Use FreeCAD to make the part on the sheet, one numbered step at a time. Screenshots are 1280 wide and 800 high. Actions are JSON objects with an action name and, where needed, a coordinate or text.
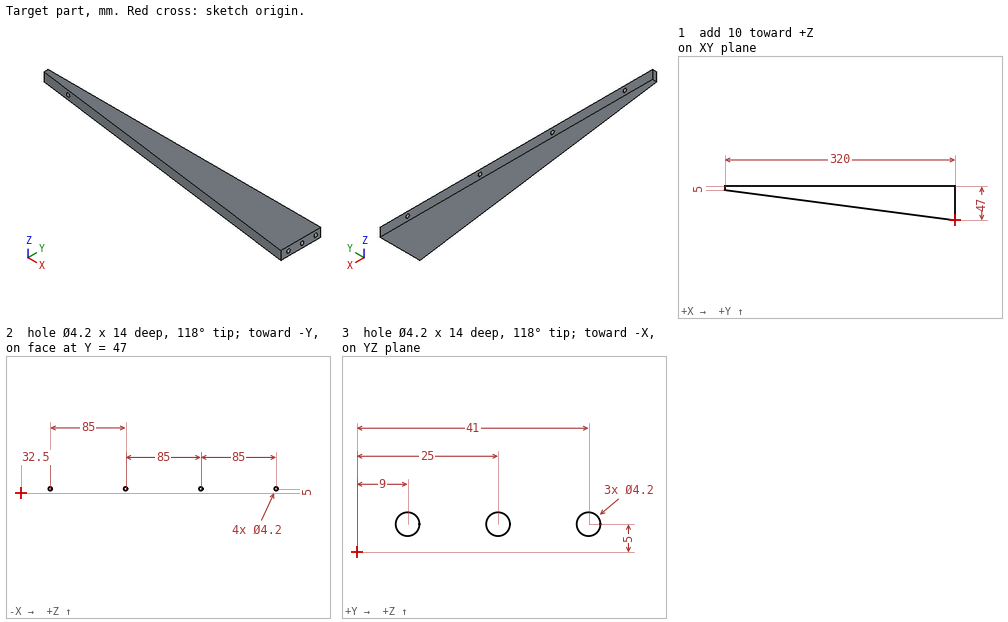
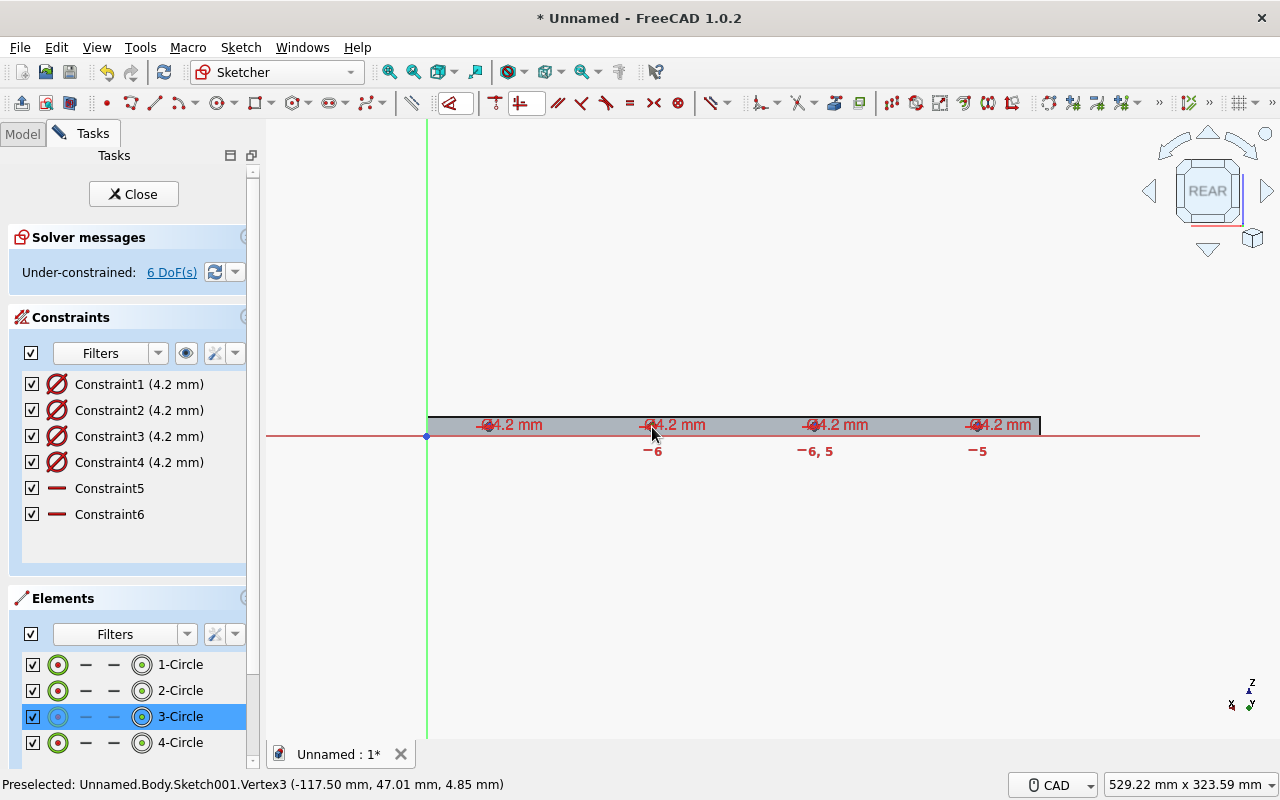
{"action": "left_click", "coordinate": [489, 427]}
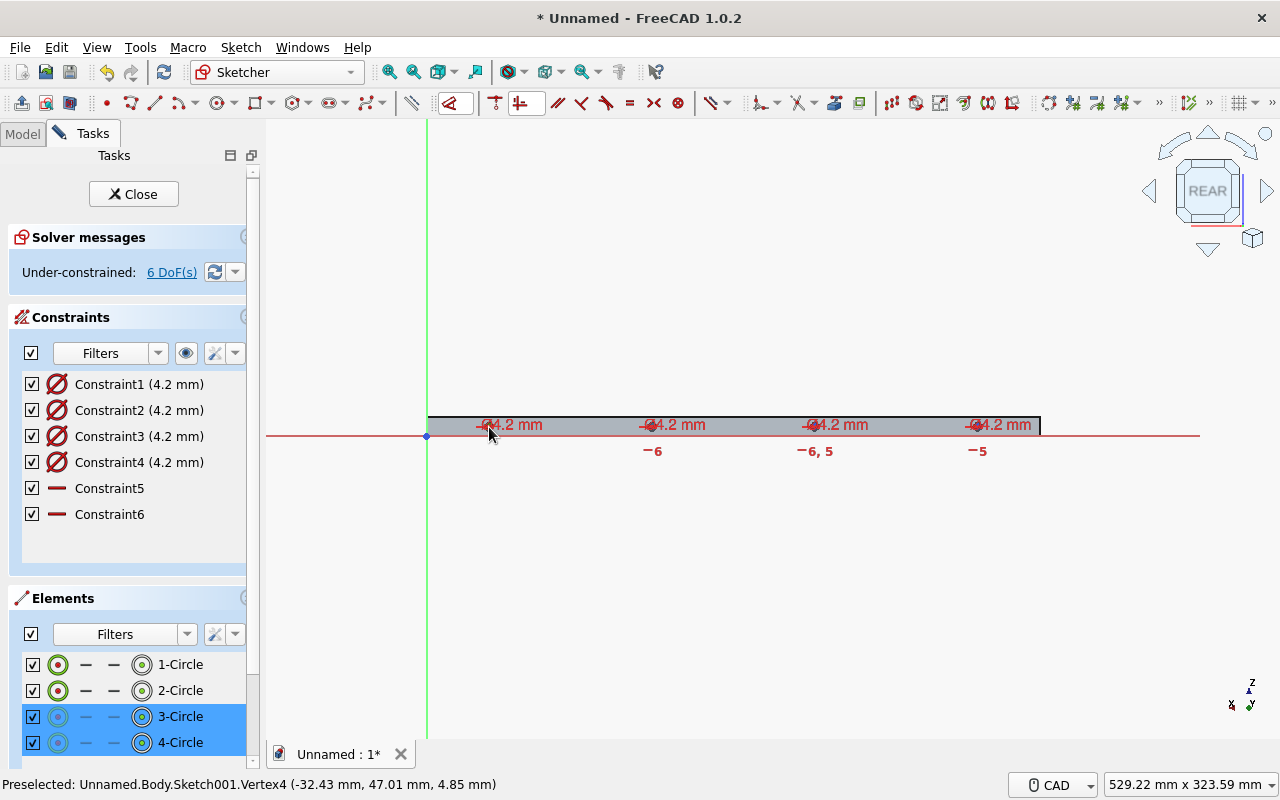
{"action": "left_click", "coordinate": [540, 104]}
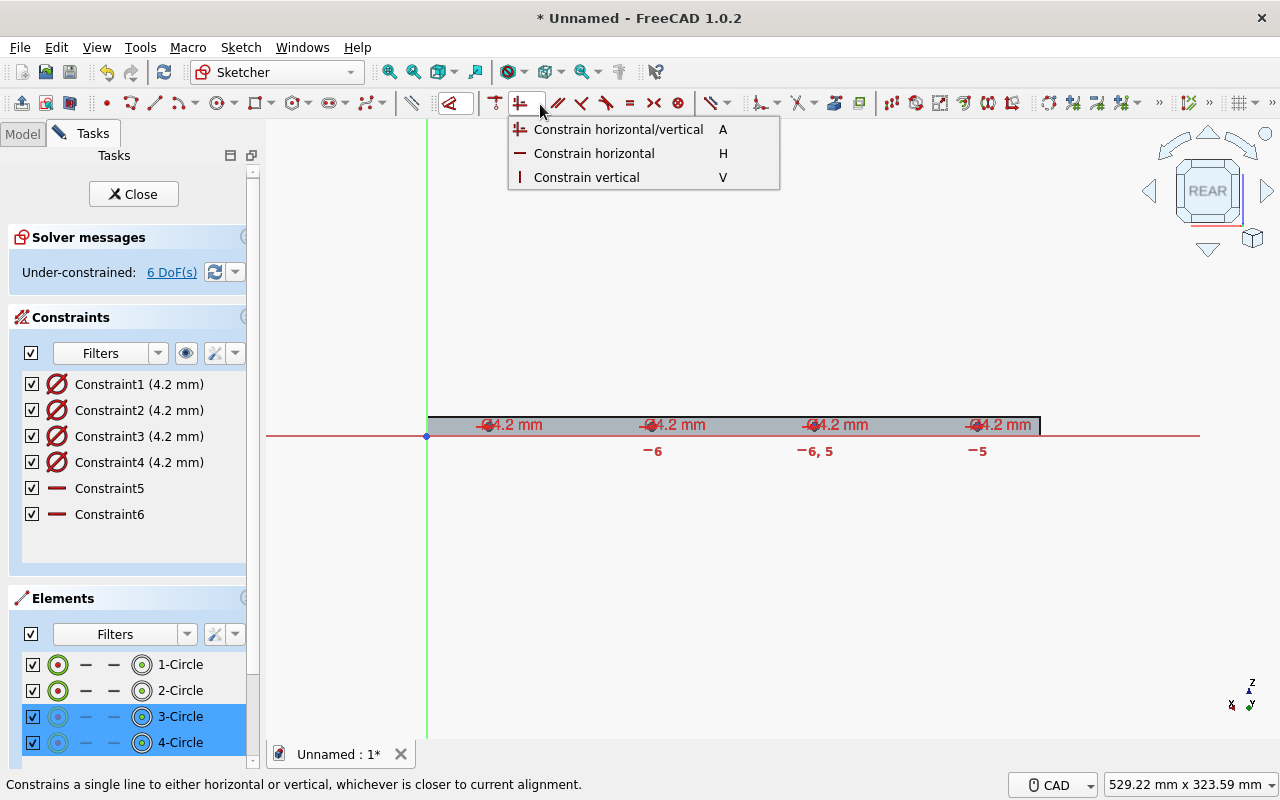
{"action": "left_click", "coordinate": [644, 153]}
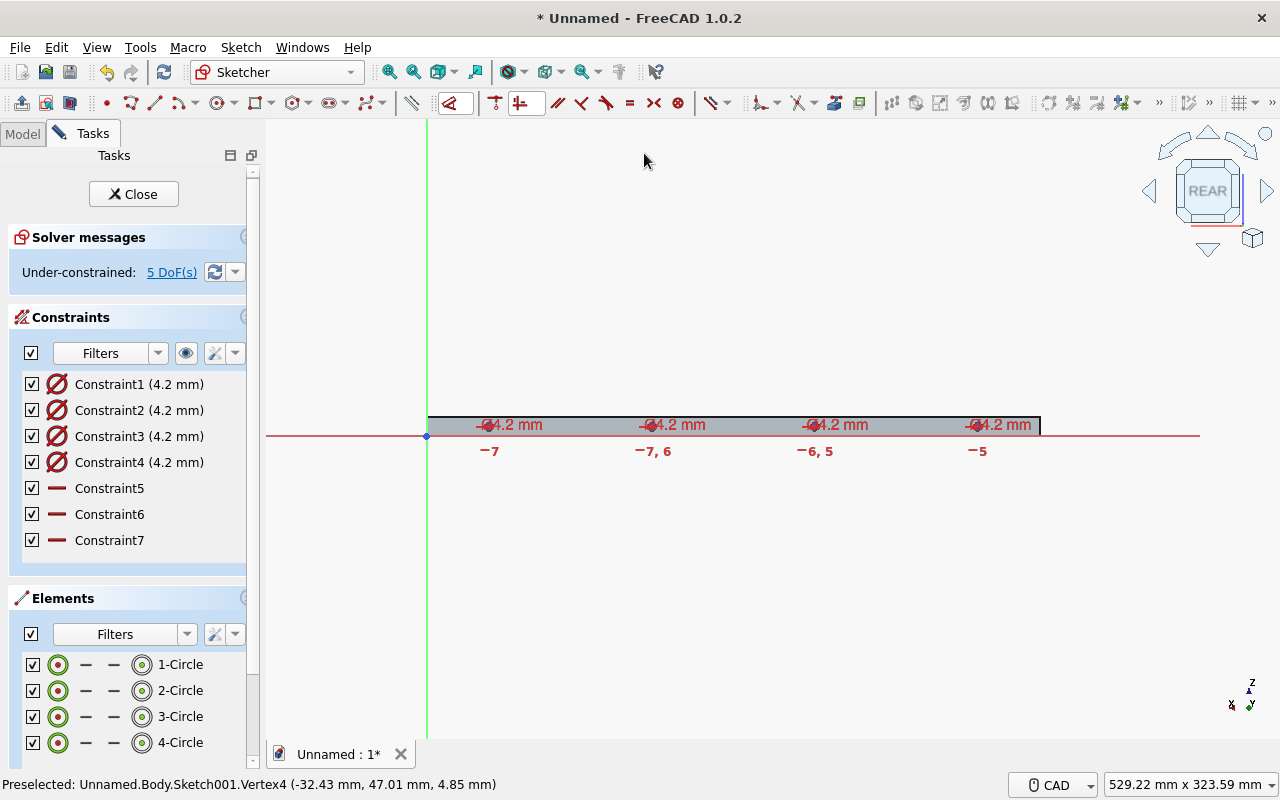
{"action": "key", "text": "d"}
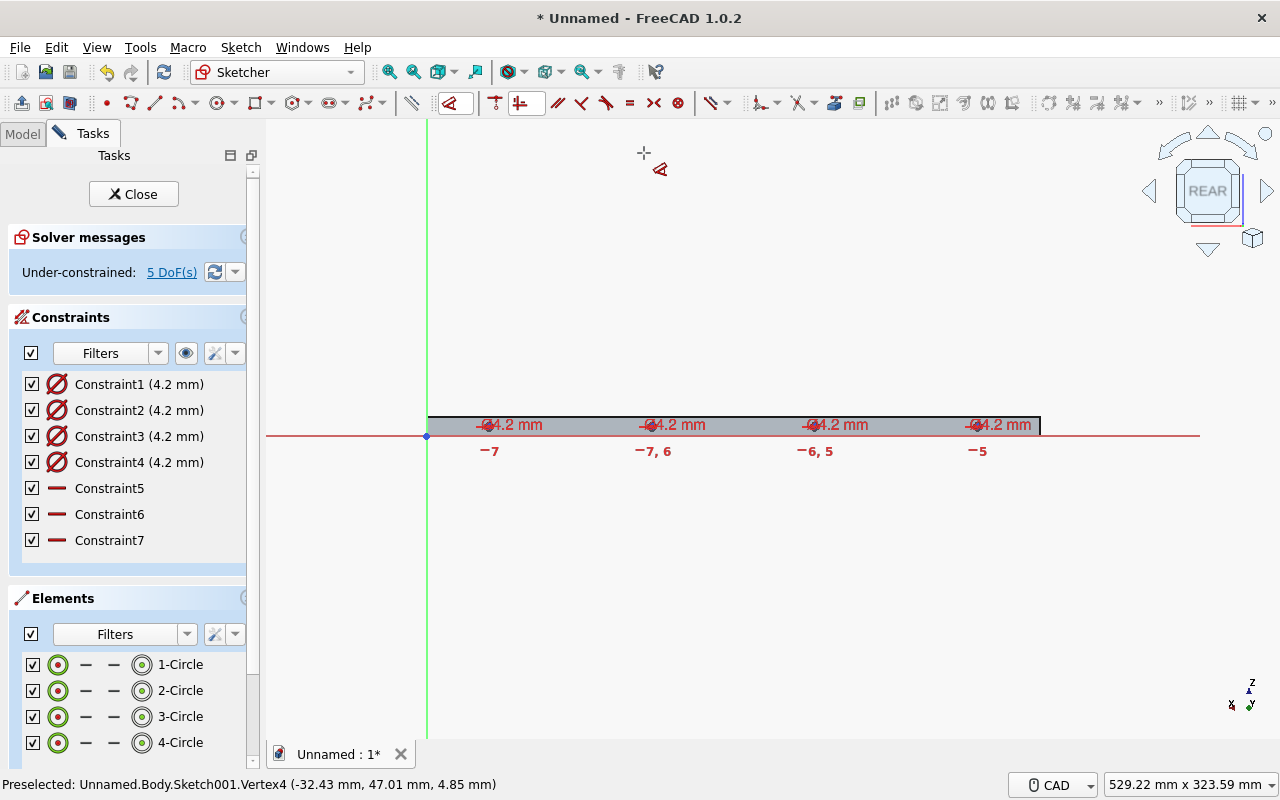
{"action": "scroll", "coordinate": [978, 427], "scroll_direction": "up", "scroll_amount": 8}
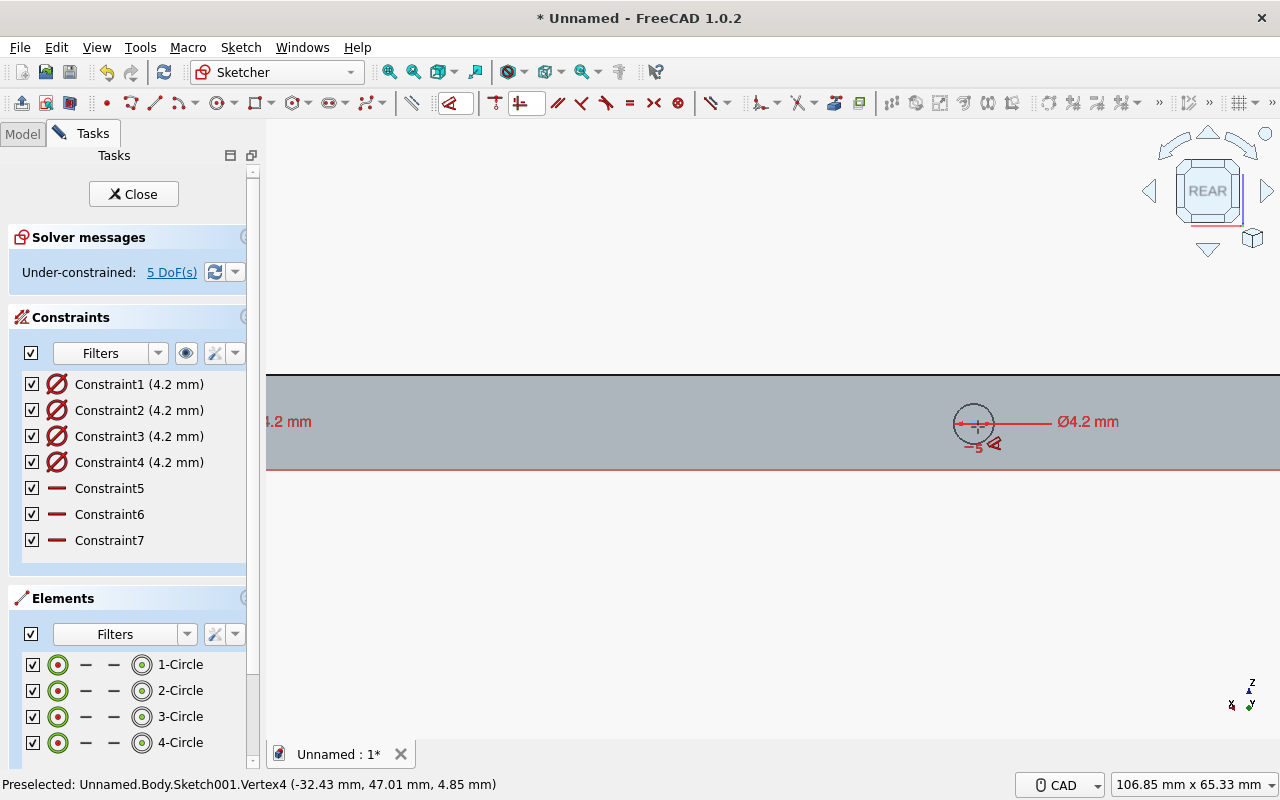
{"action": "left_click", "coordinate": [974, 424]}
{"action": "left_click", "coordinate": [1008, 447]}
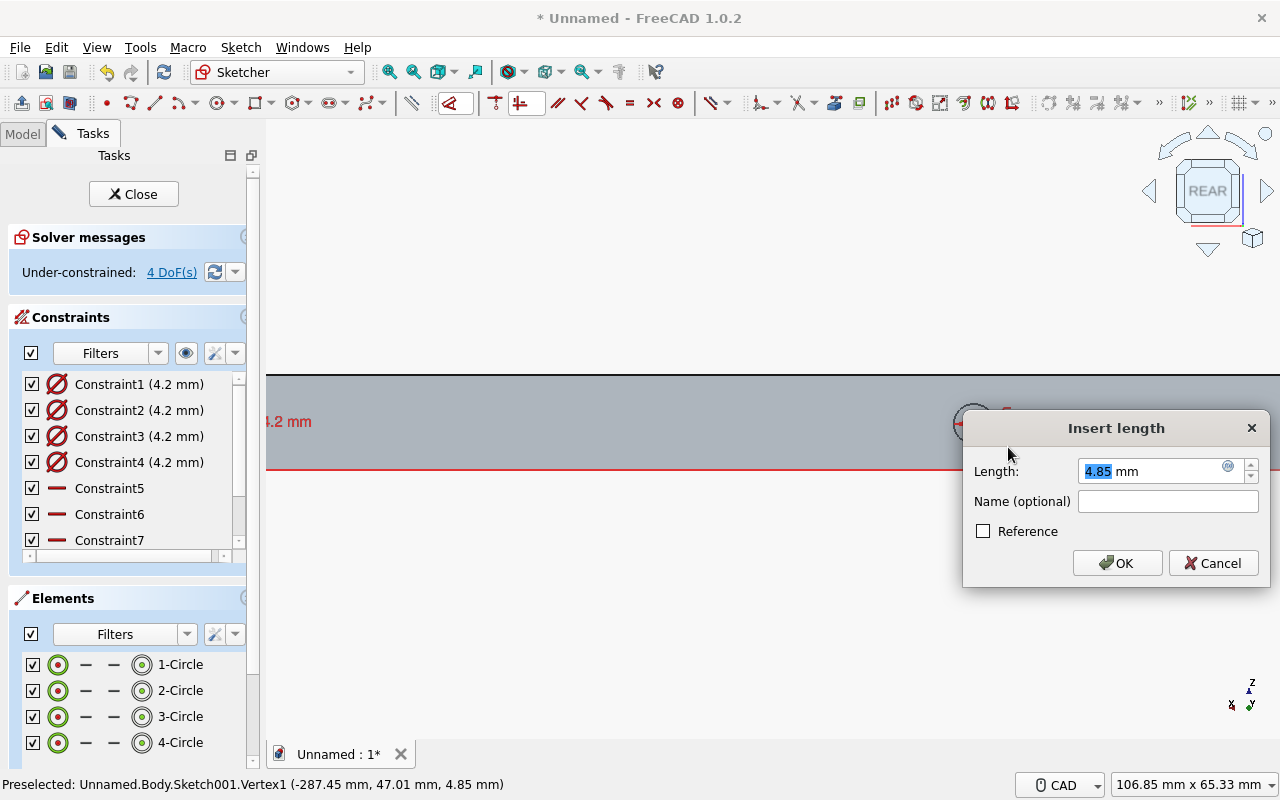
{"action": "type", "text": "5"}
{"action": "key", "text": "Return"}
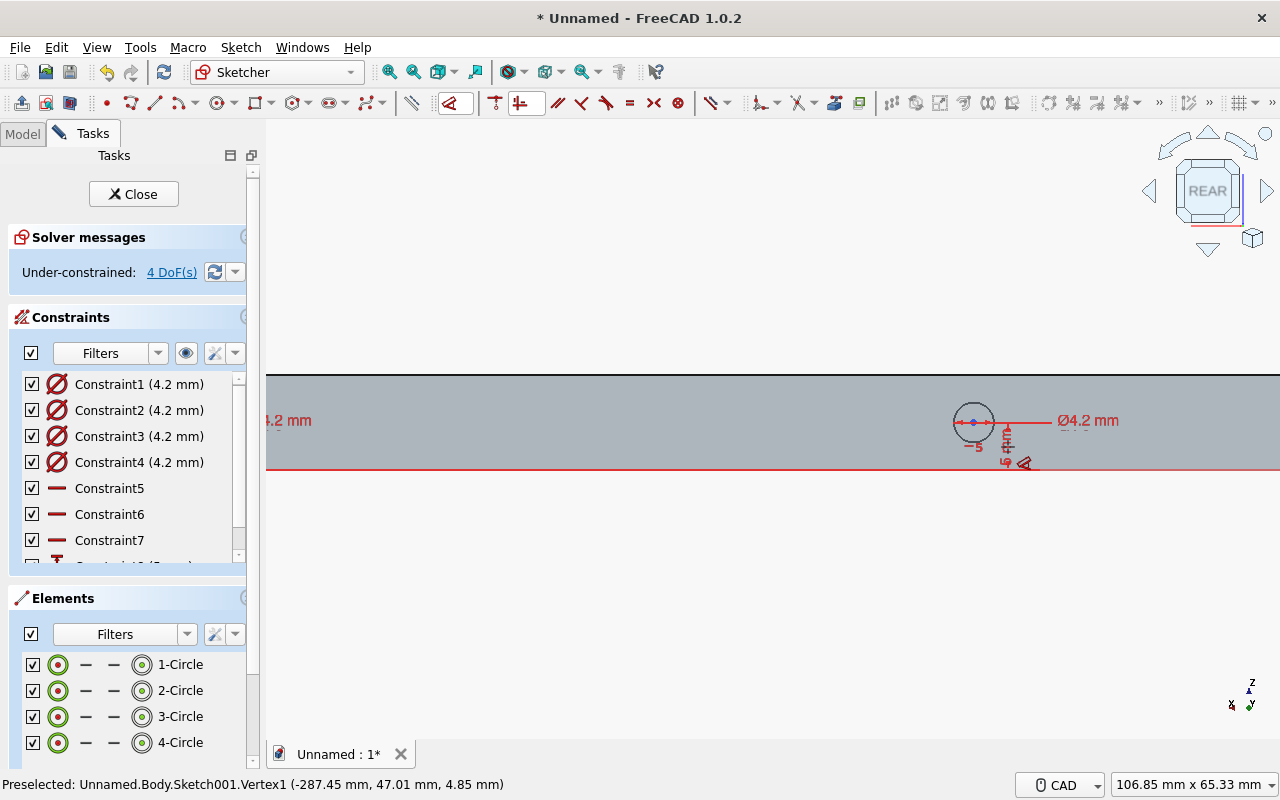
{"action": "scroll", "coordinate": [979, 427], "scroll_direction": "down", "scroll_amount": 8}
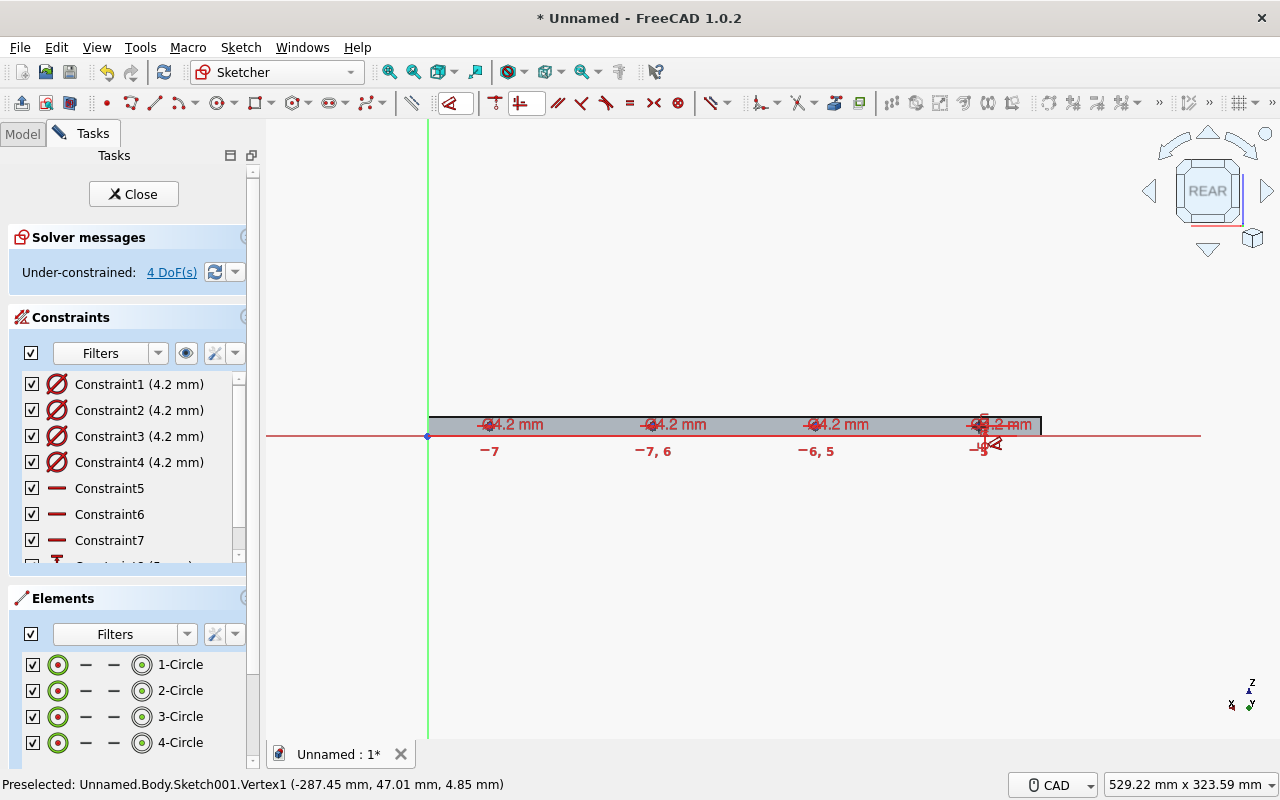
{"action": "left_click", "coordinate": [979, 426]}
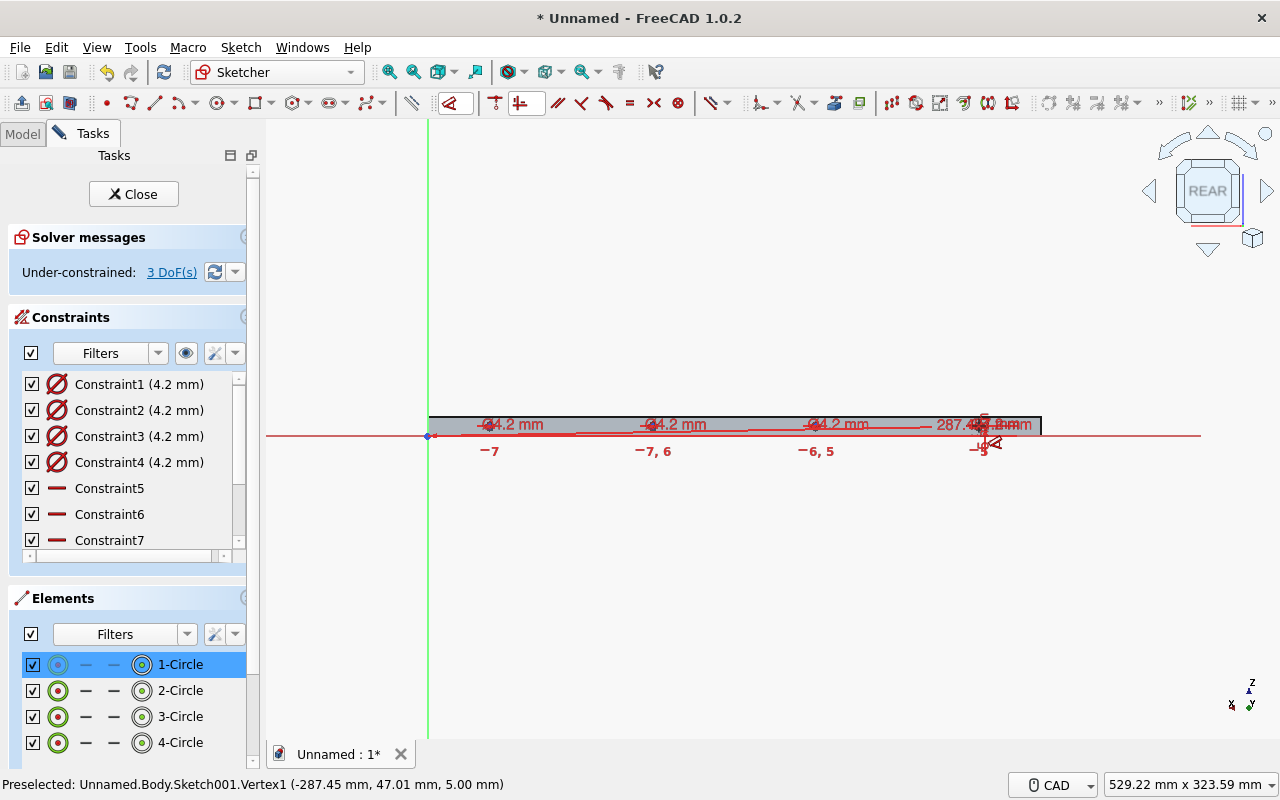
{"action": "left_click", "coordinate": [816, 426]}
{"action": "left_click", "coordinate": [897, 392]}